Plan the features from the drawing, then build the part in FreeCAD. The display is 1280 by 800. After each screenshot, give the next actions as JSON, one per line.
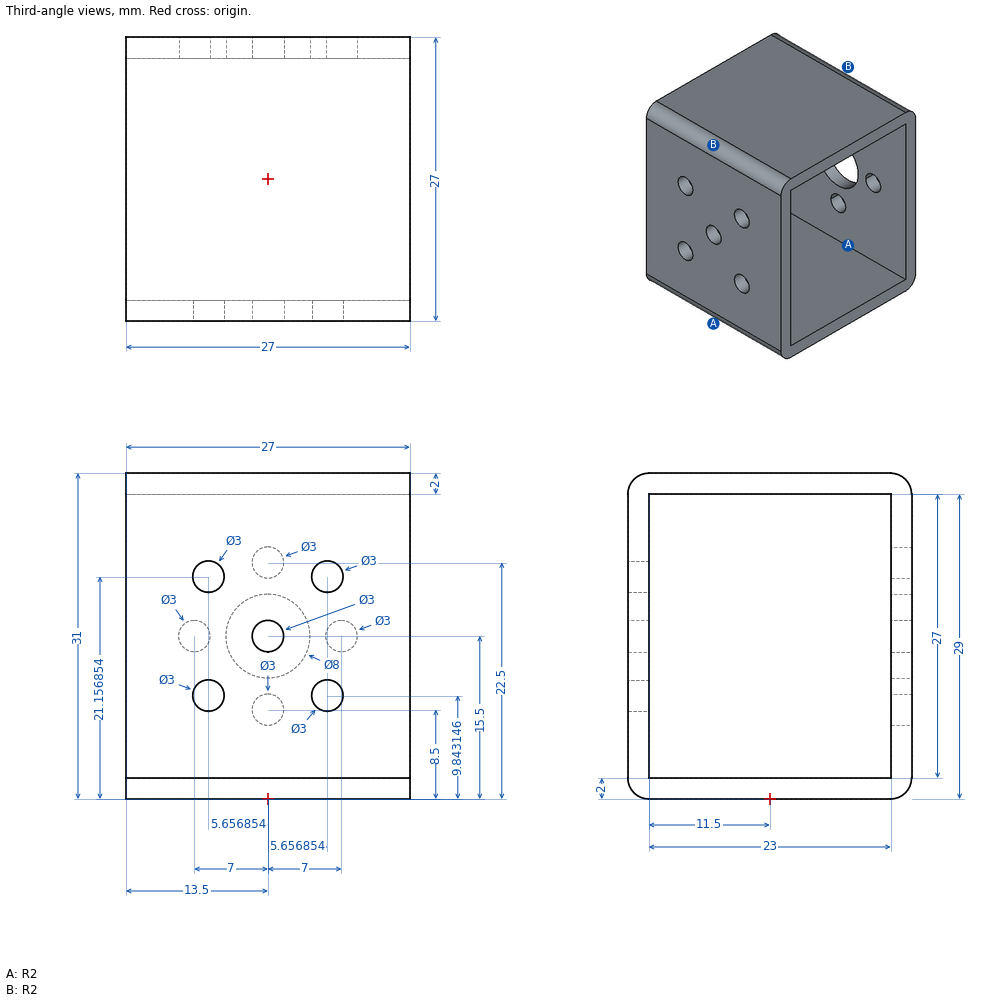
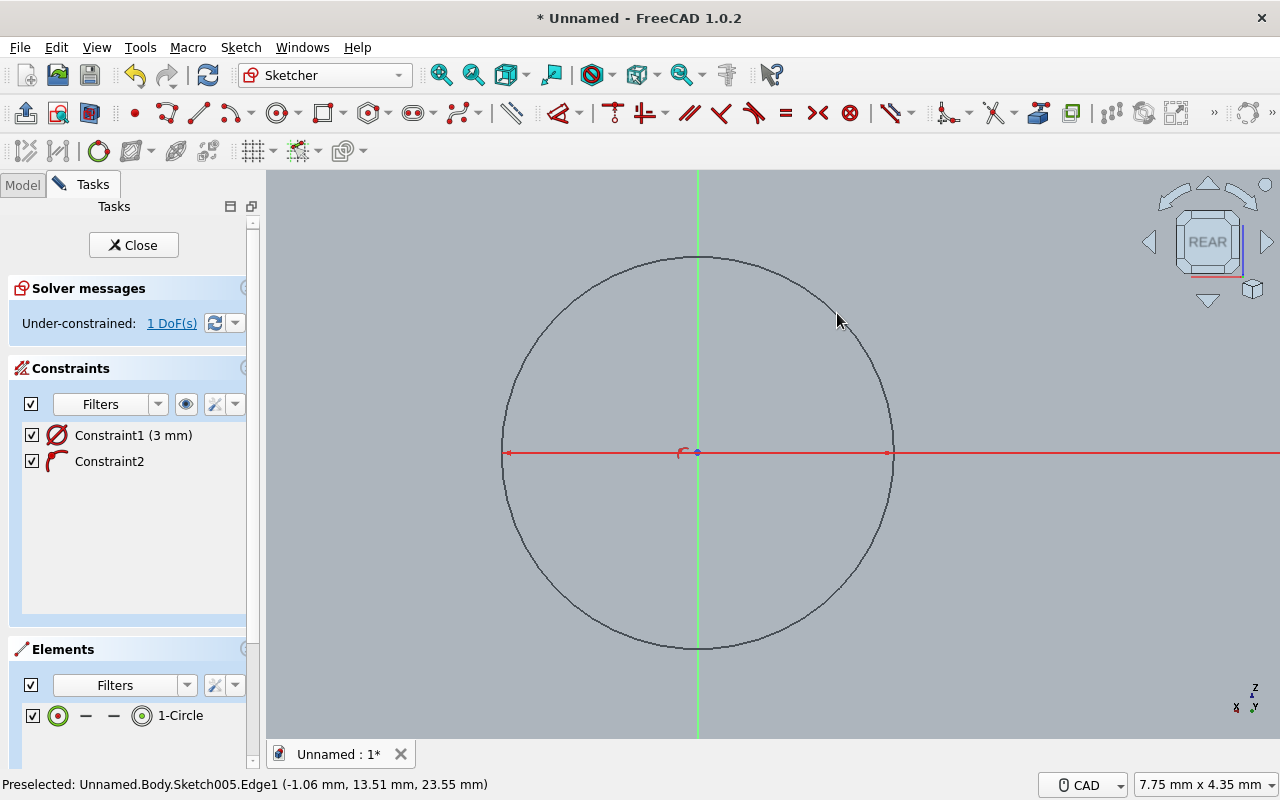
{"action": "left_click", "coordinate": [558, 114]}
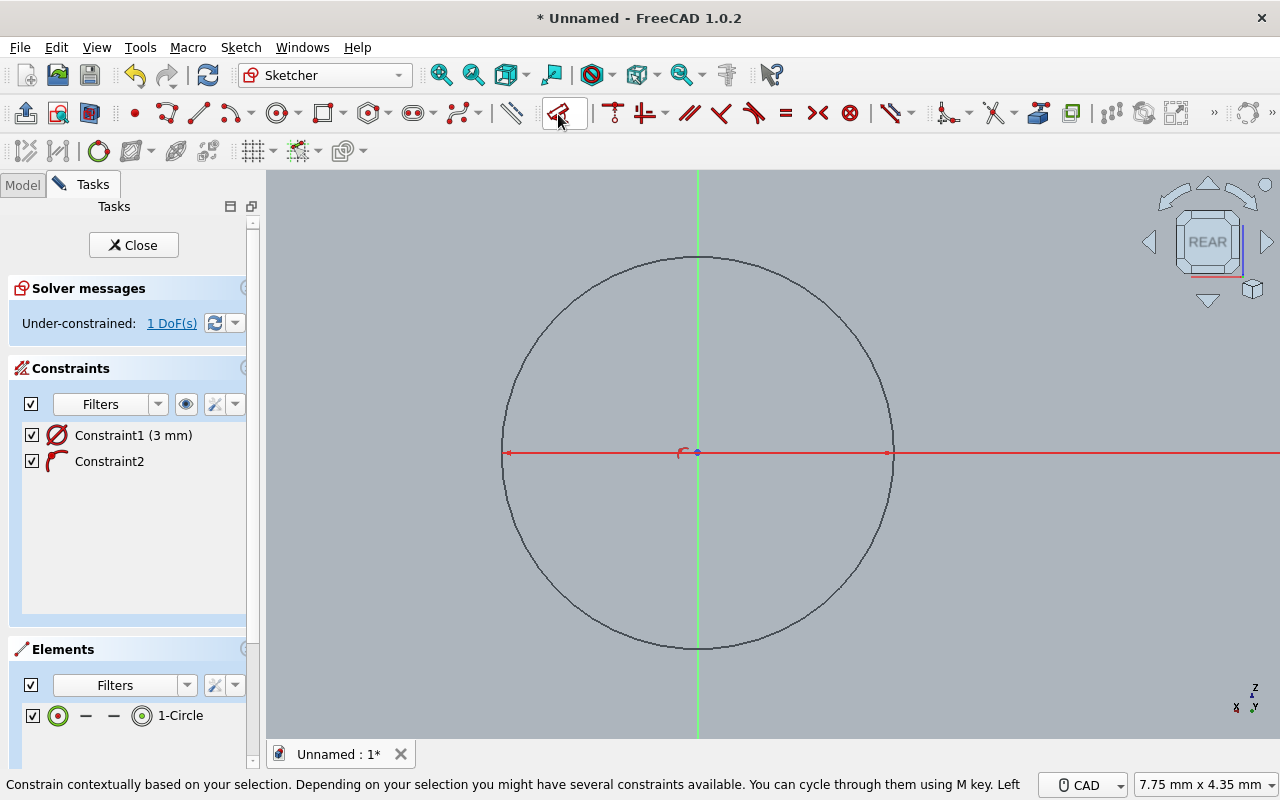
{"action": "left_click", "coordinate": [698, 453]}
{"action": "left_click", "coordinate": [732, 582]}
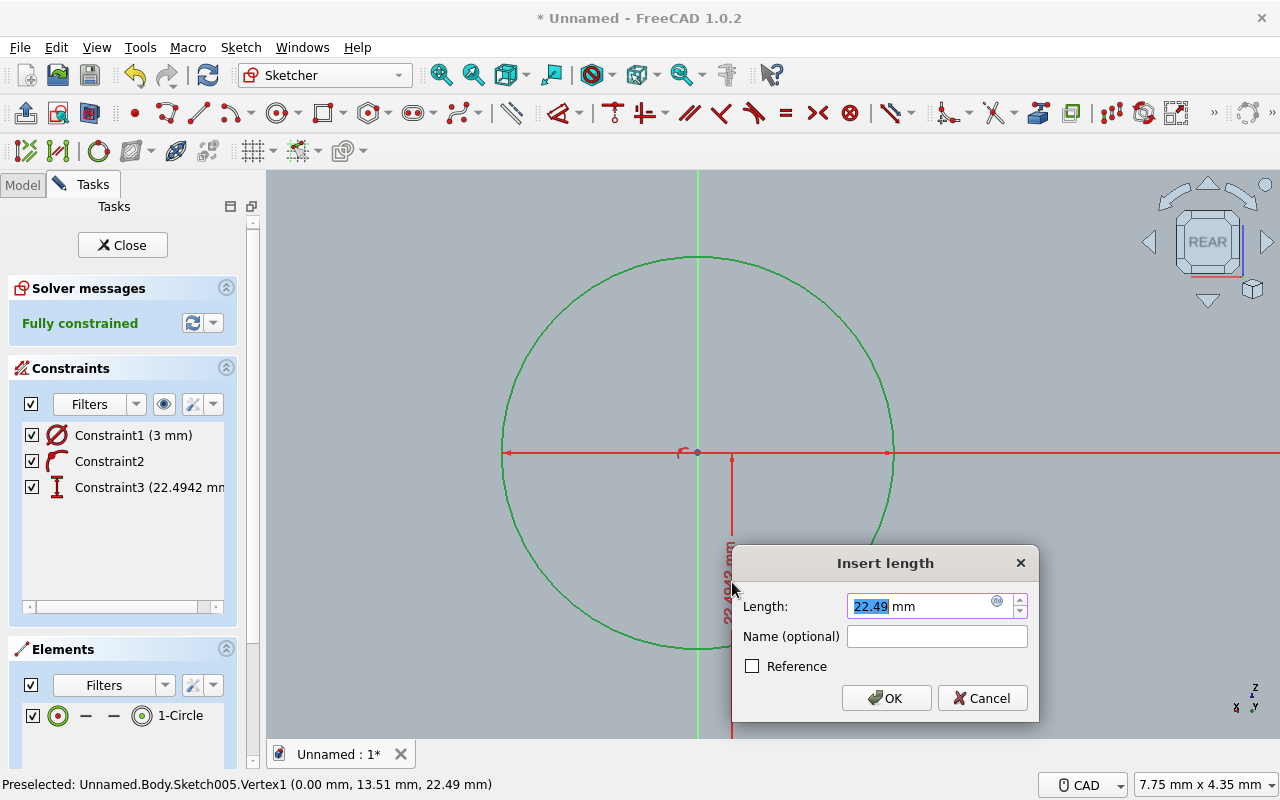
{"action": "type", "text": "22.5"}
{"action": "key", "text": "Return"}
{"action": "key", "text": "Escape"}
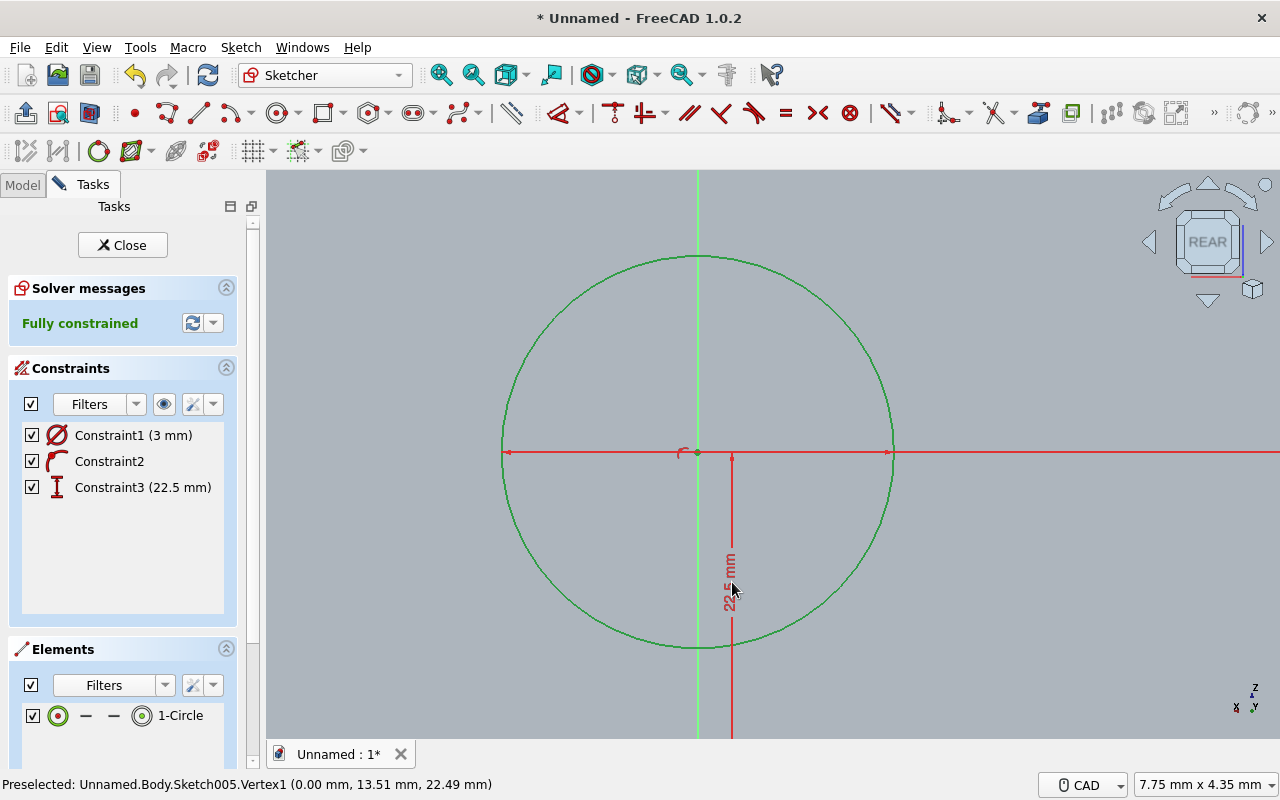
{"action": "left_click", "coordinate": [123, 245]}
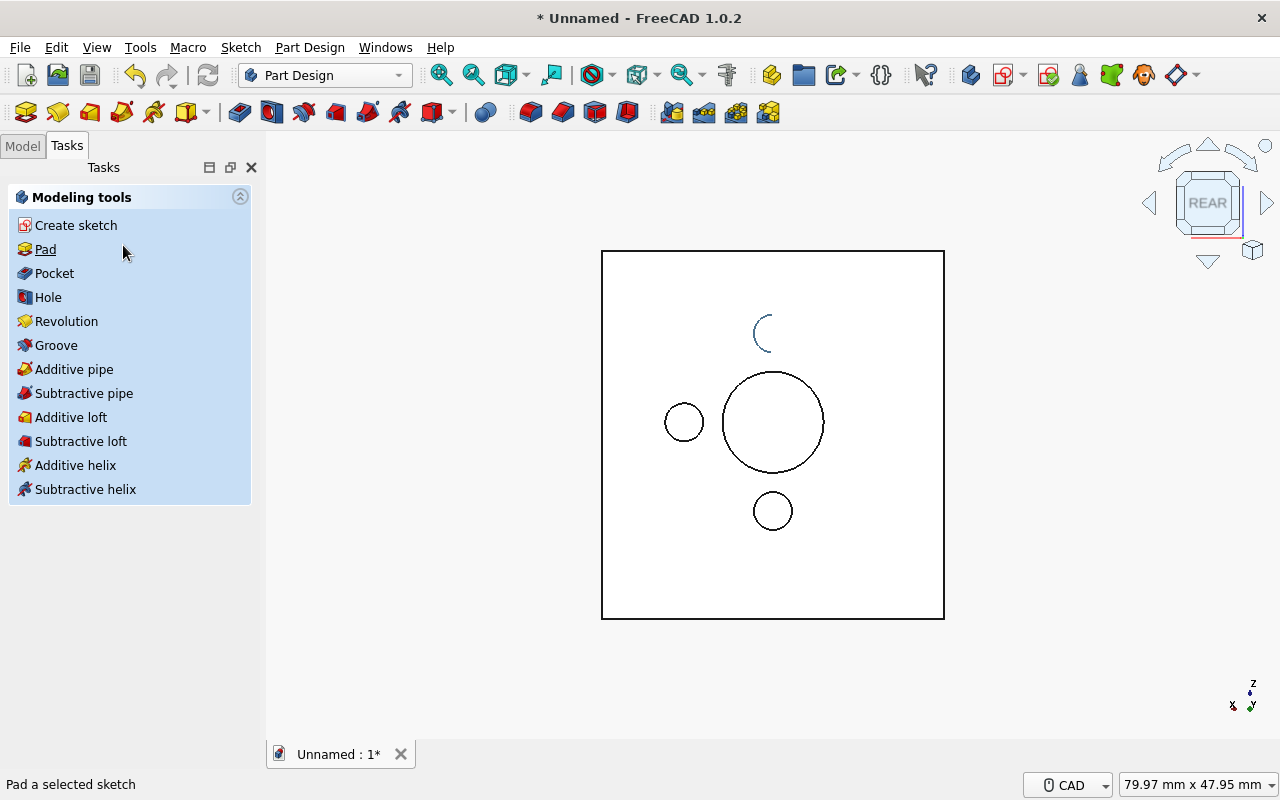
{"action": "left_click", "coordinate": [240, 112]}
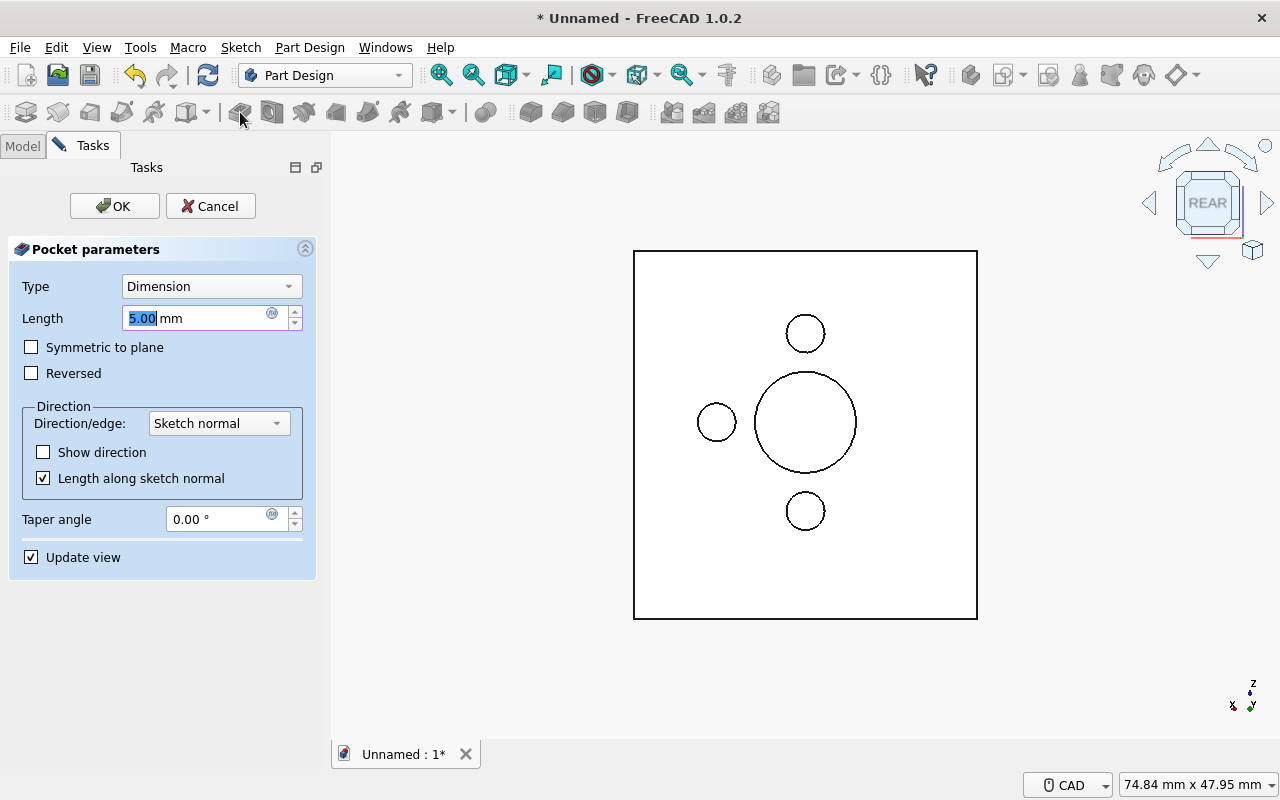
{"action": "left_click", "coordinate": [212, 286]}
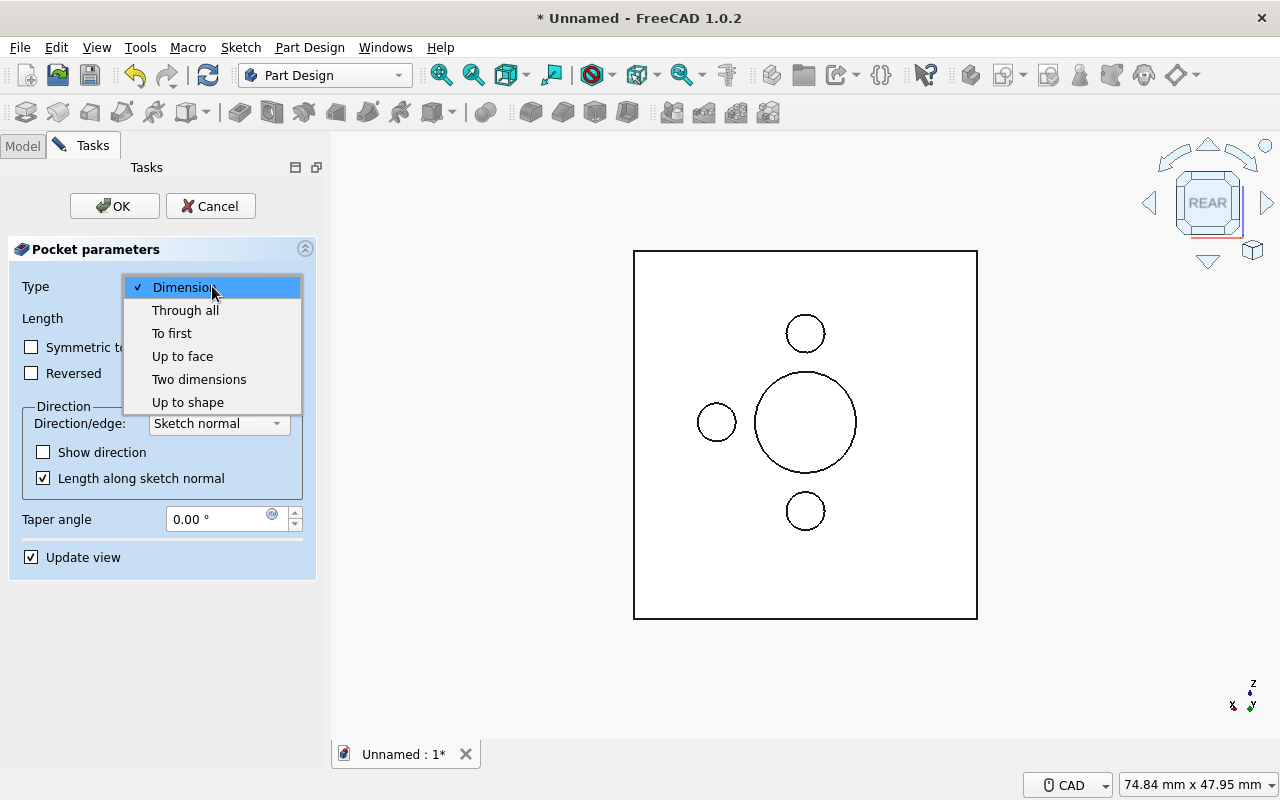
{"action": "left_click", "coordinate": [212, 334]}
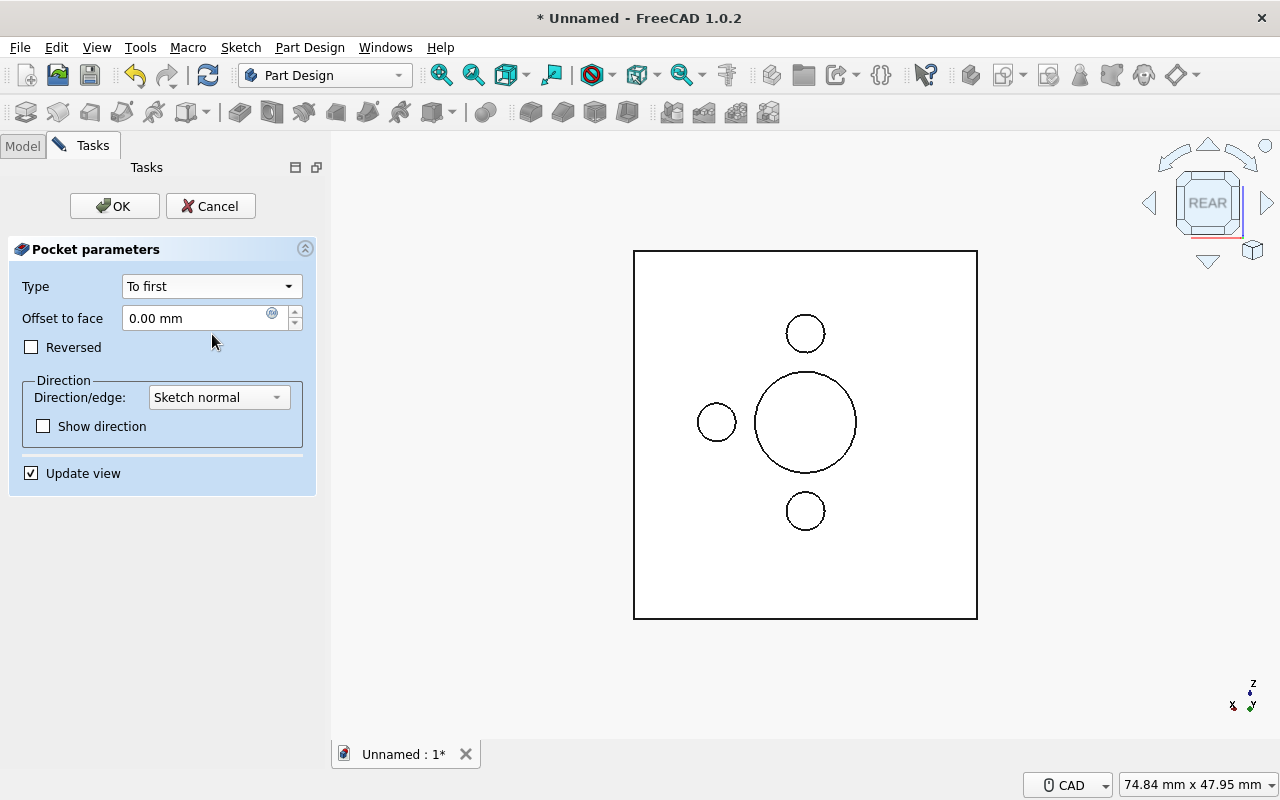
{"action": "left_click", "coordinate": [115, 206]}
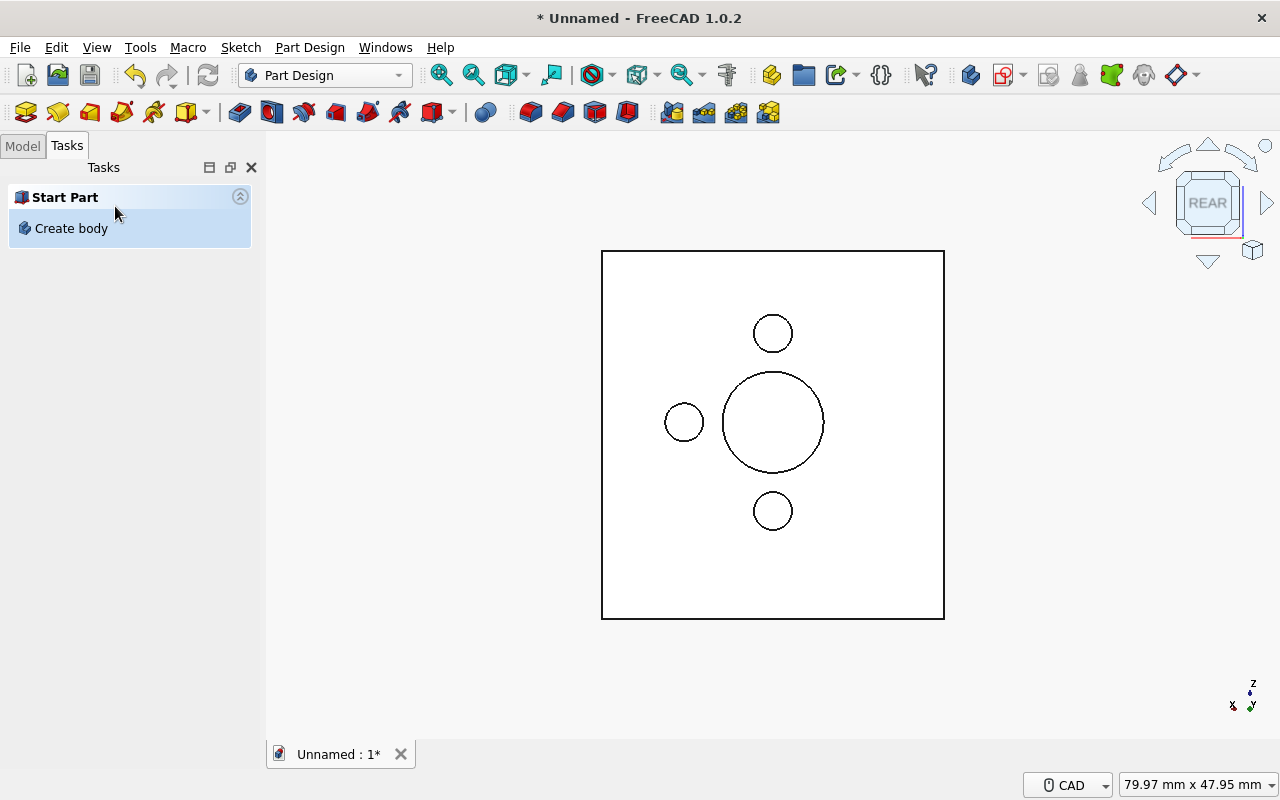
{"action": "left_click", "coordinate": [675, 329]}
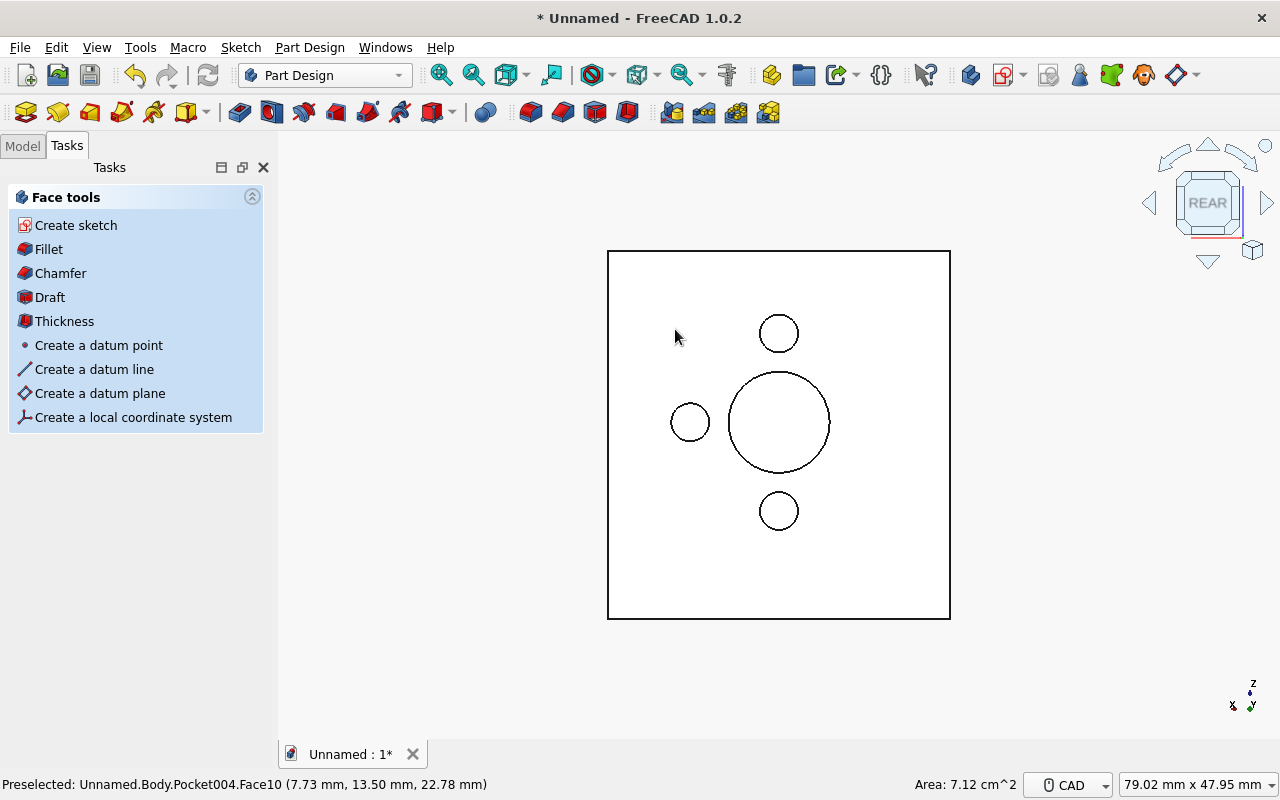
{"action": "left_click", "coordinate": [1004, 76]}